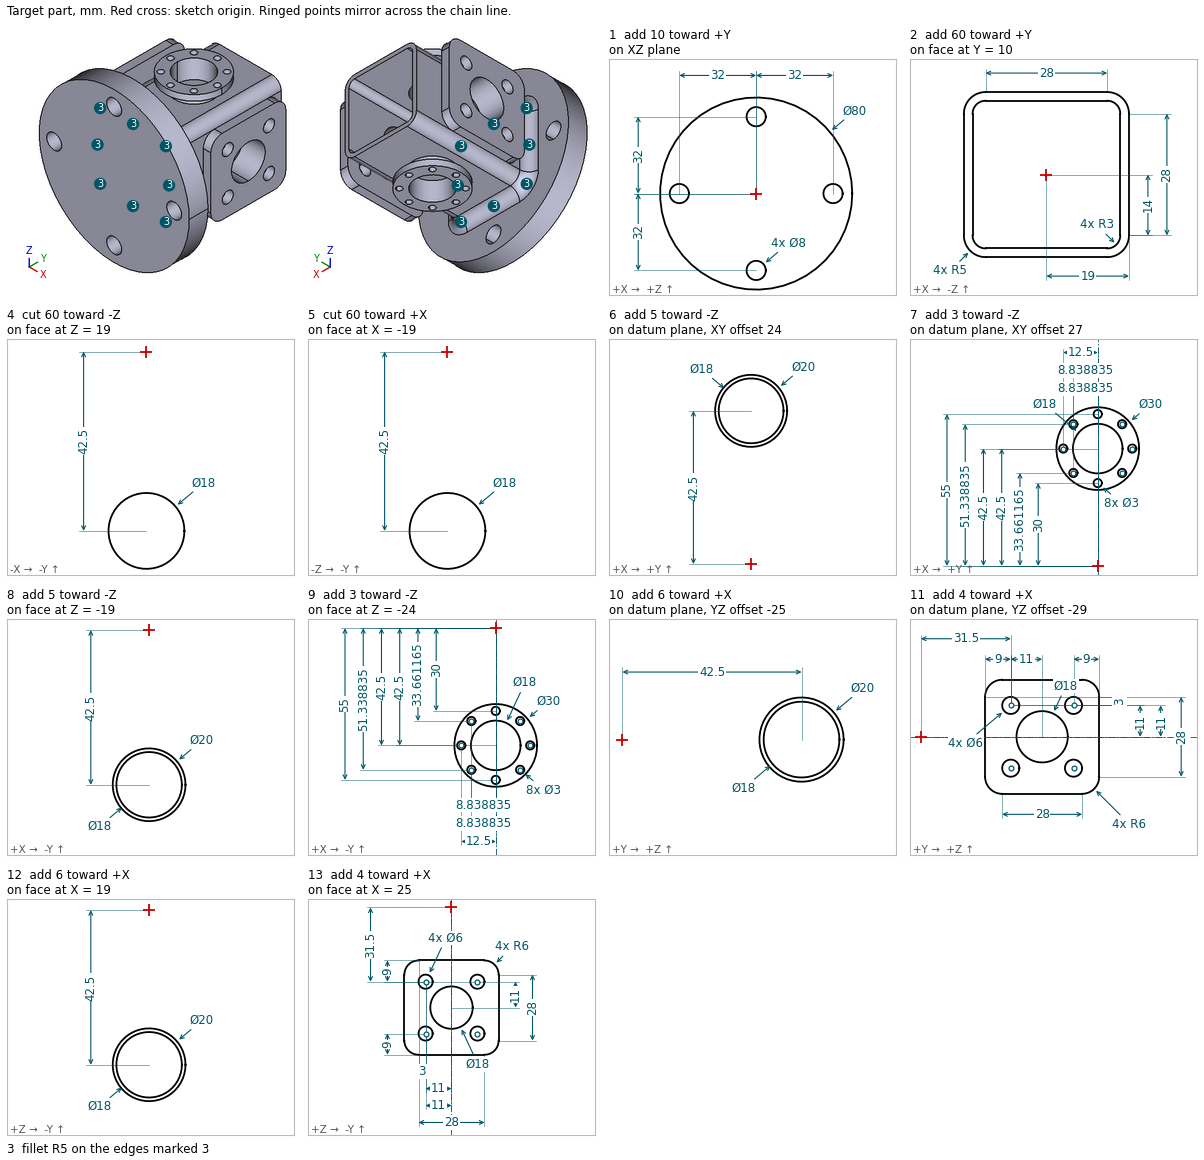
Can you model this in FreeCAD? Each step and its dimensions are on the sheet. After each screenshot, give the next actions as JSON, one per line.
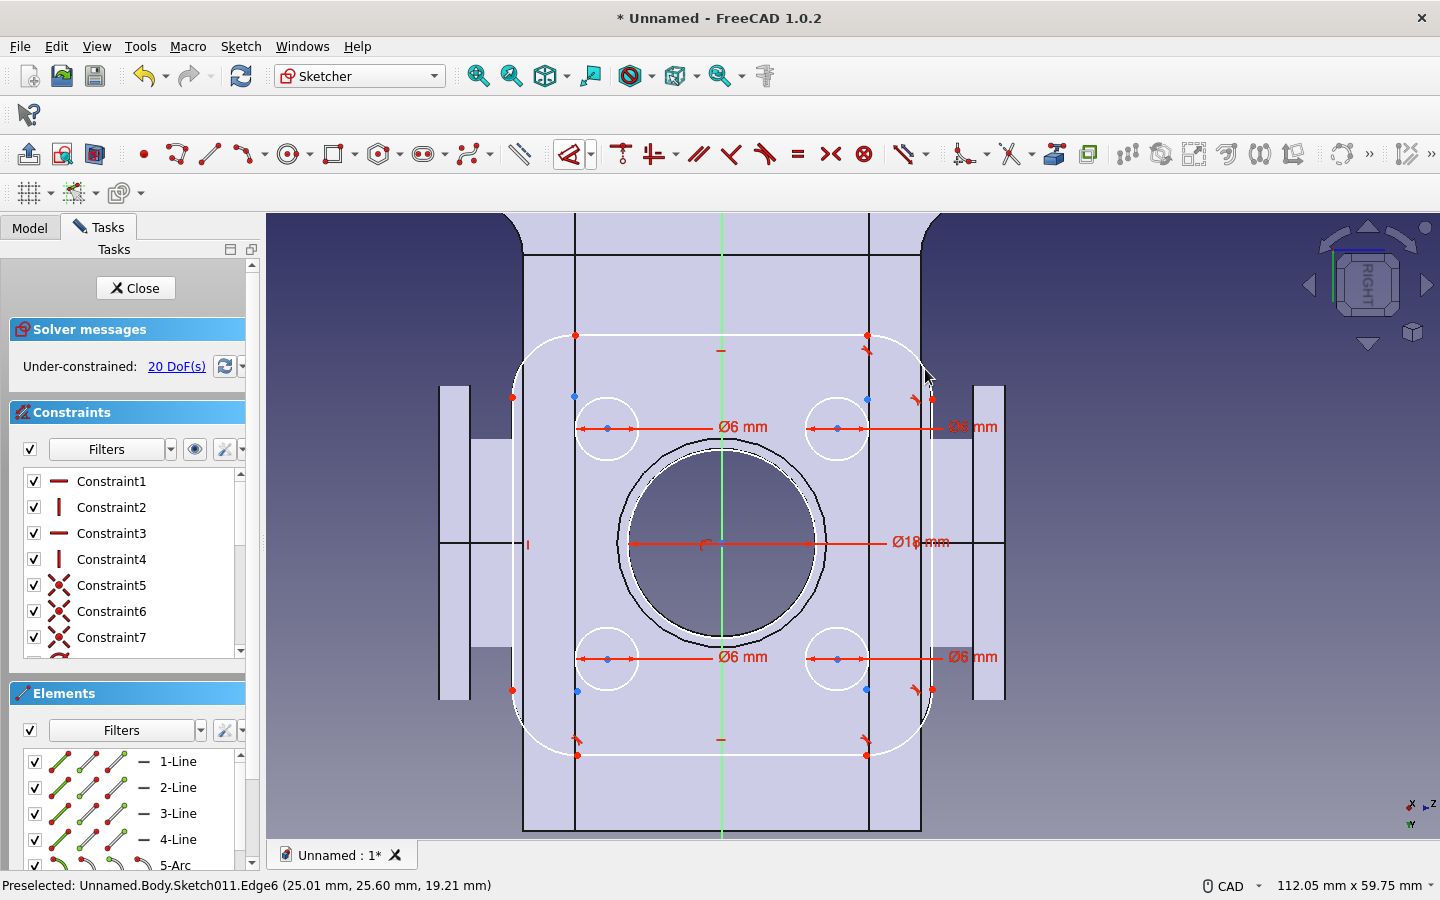
{"action": "left_click", "coordinate": [780, 335]}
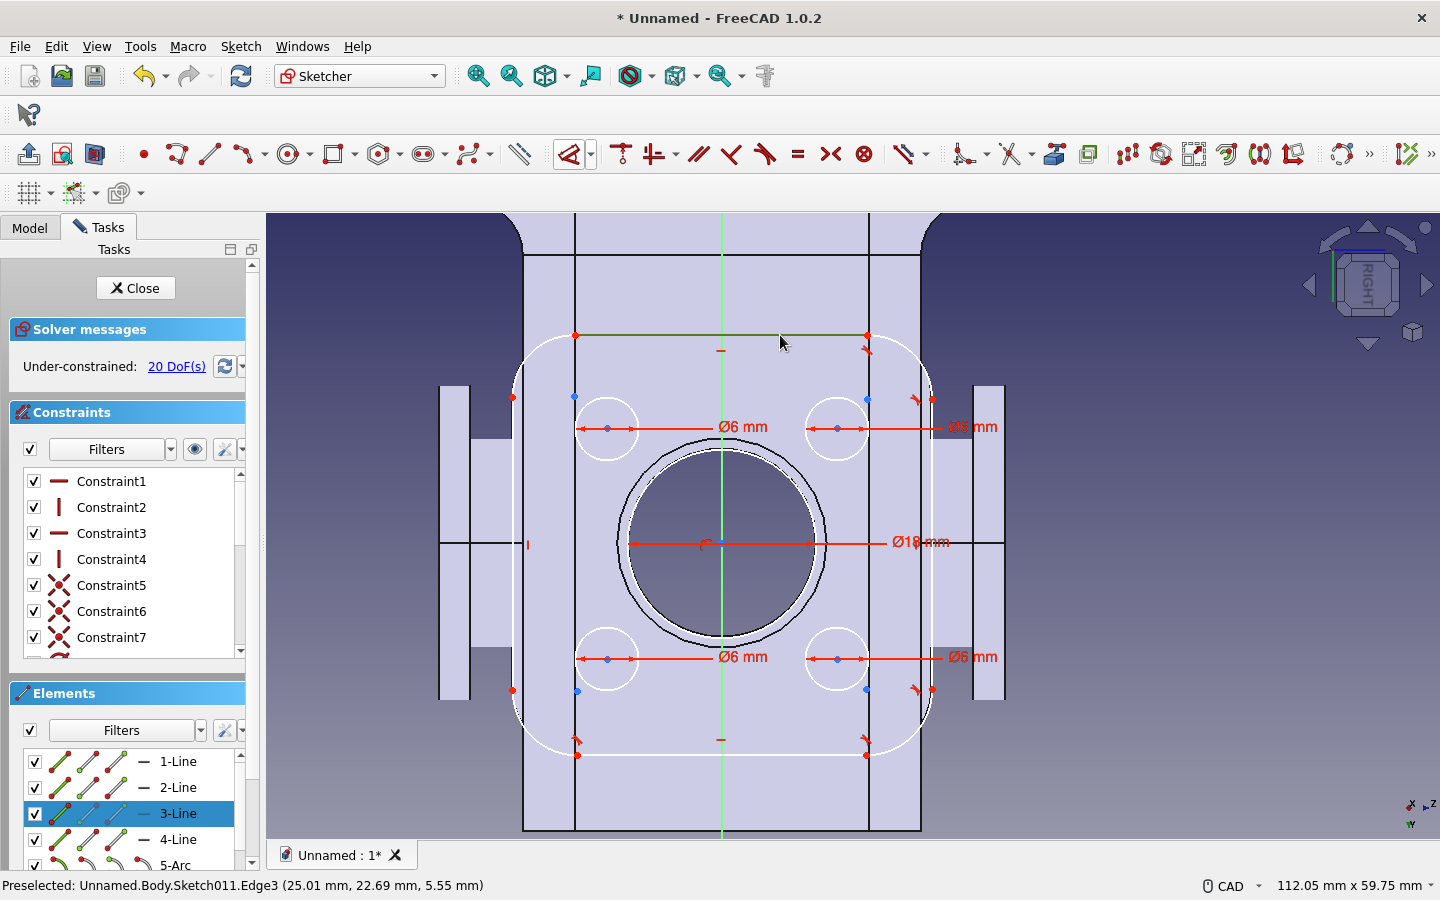
{"action": "left_click", "coordinate": [547, 342]}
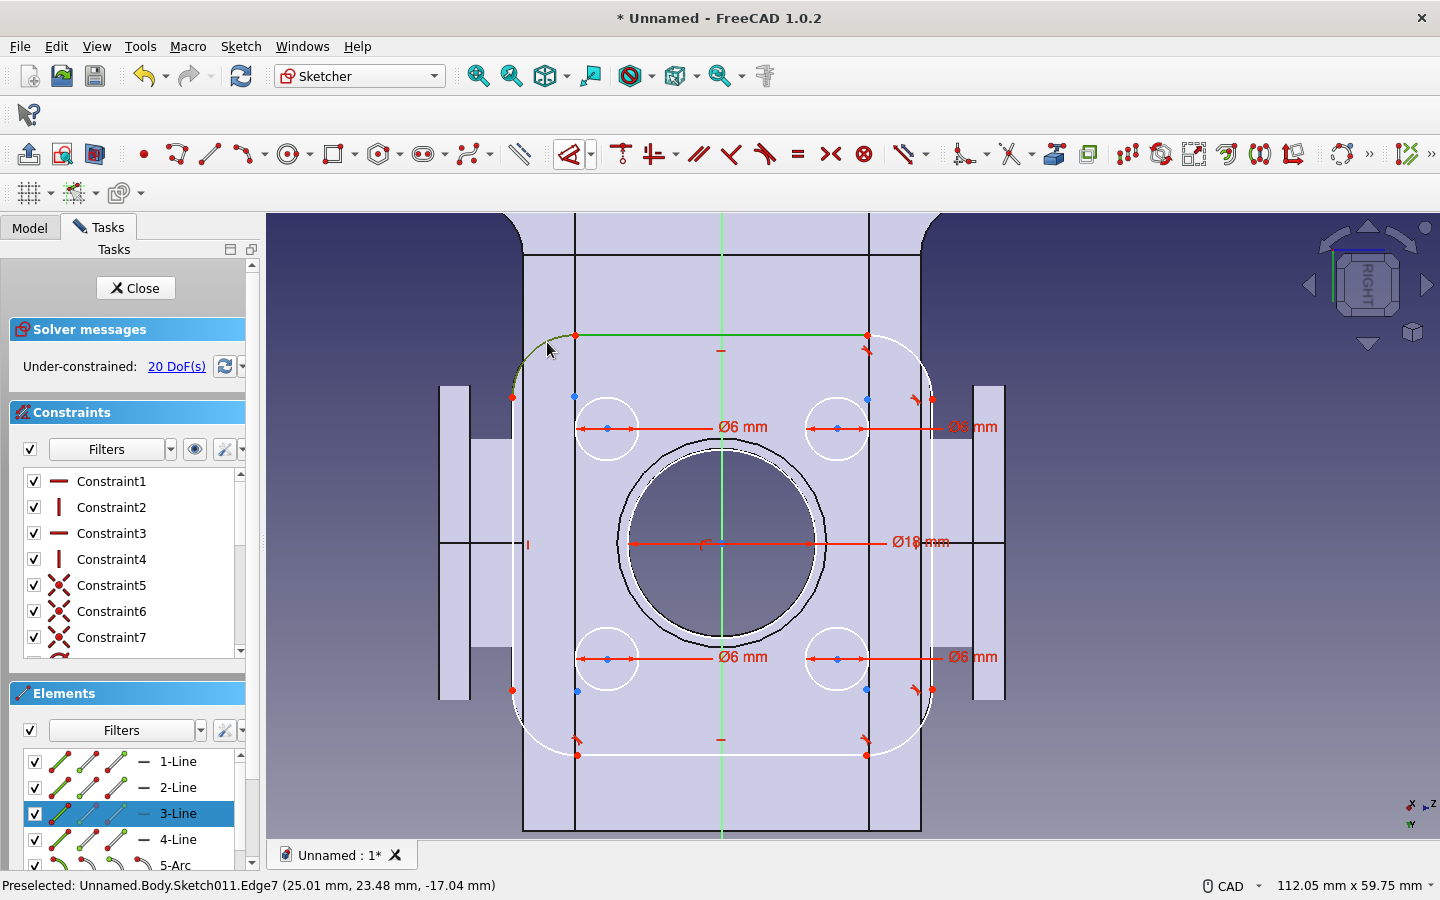
{"action": "key", "text": "t"}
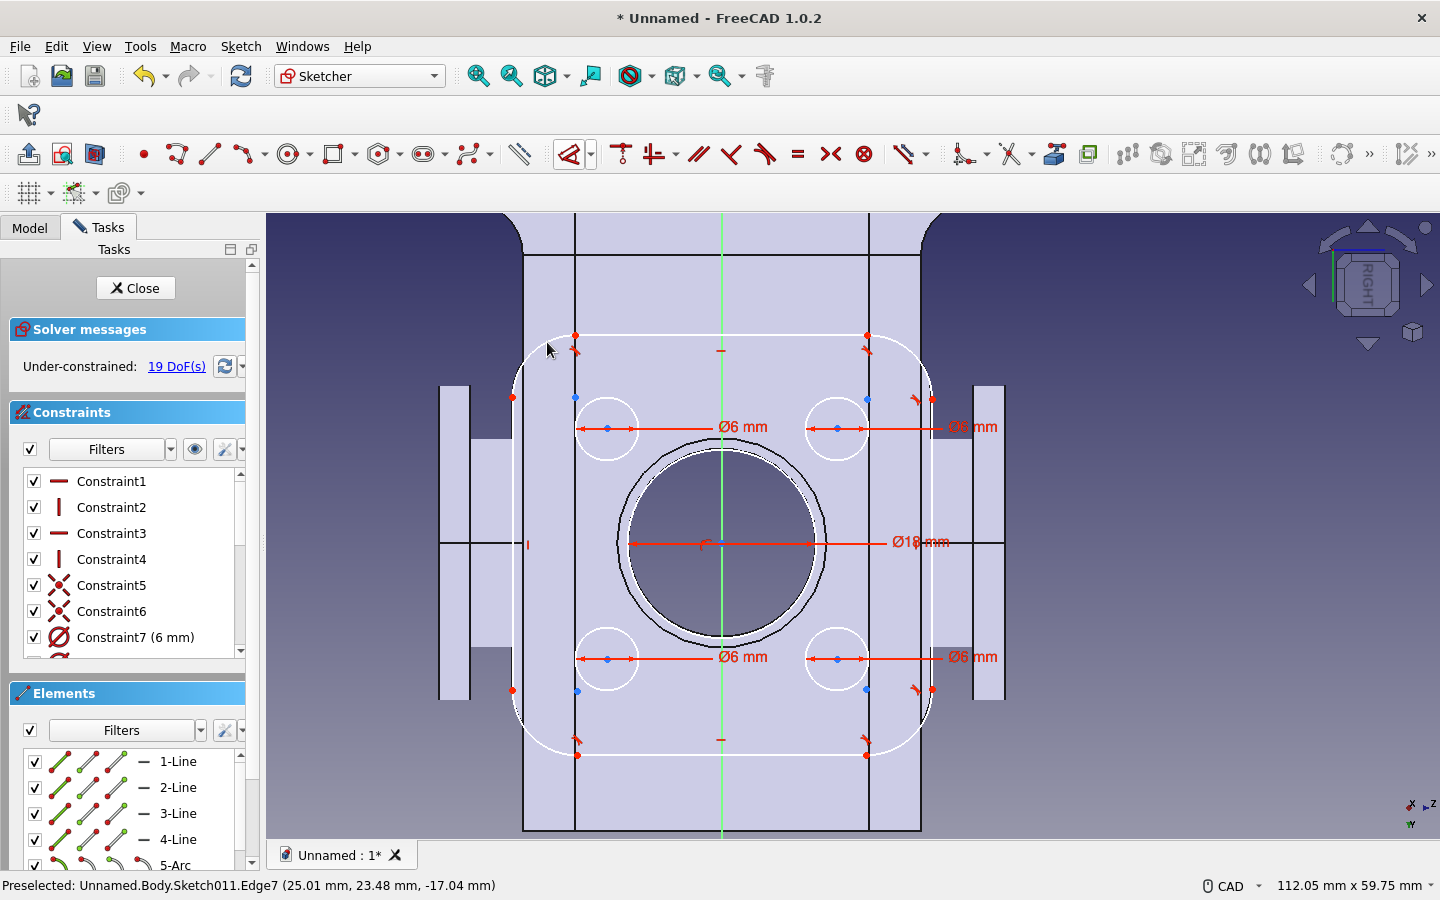
{"action": "left_click", "coordinate": [513, 486]}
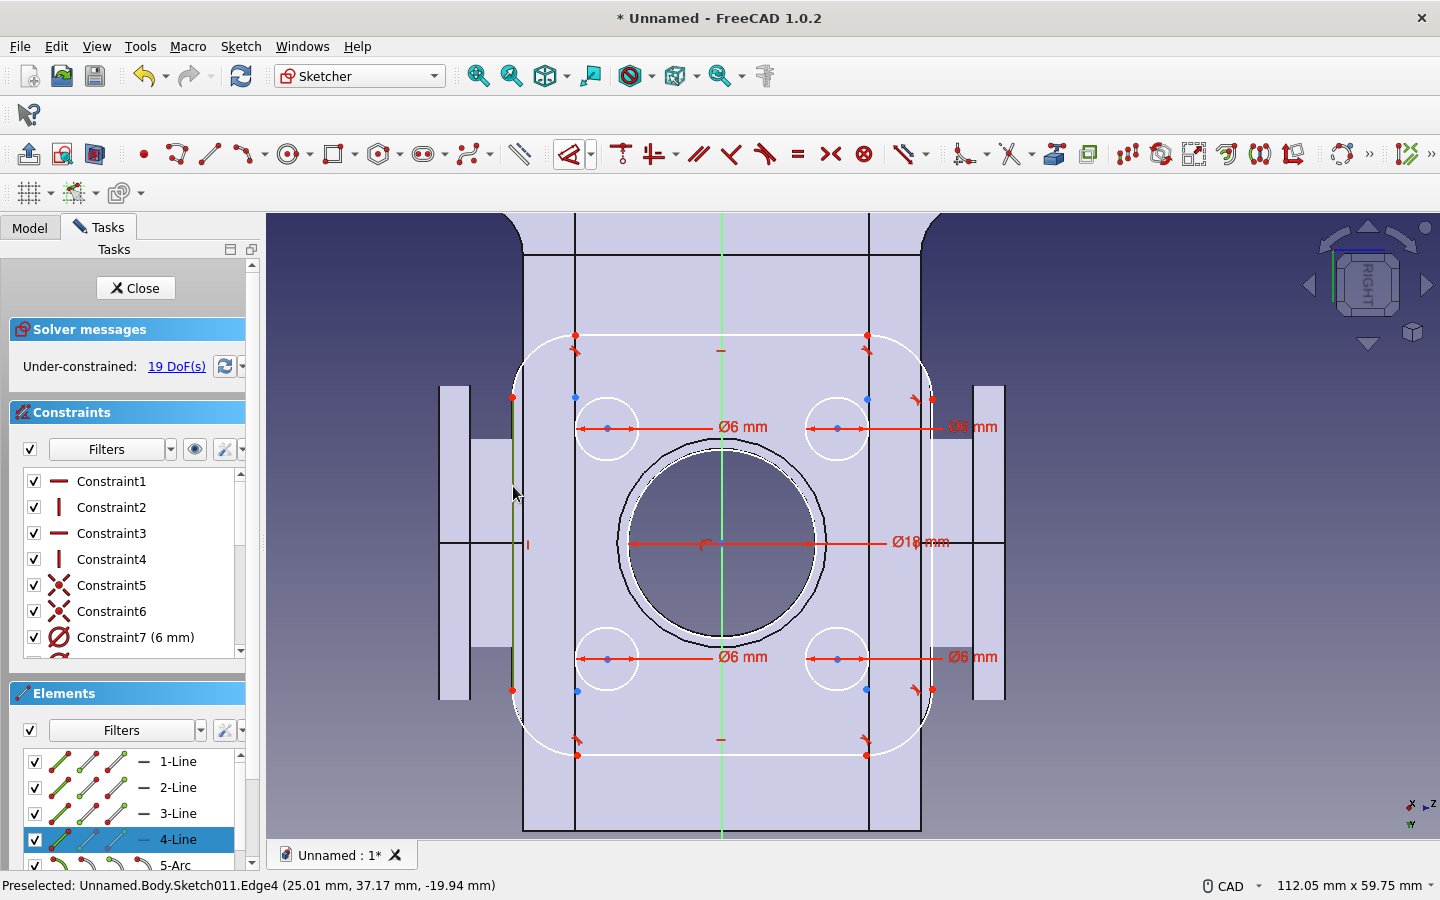
{"action": "left_click", "coordinate": [547, 342]}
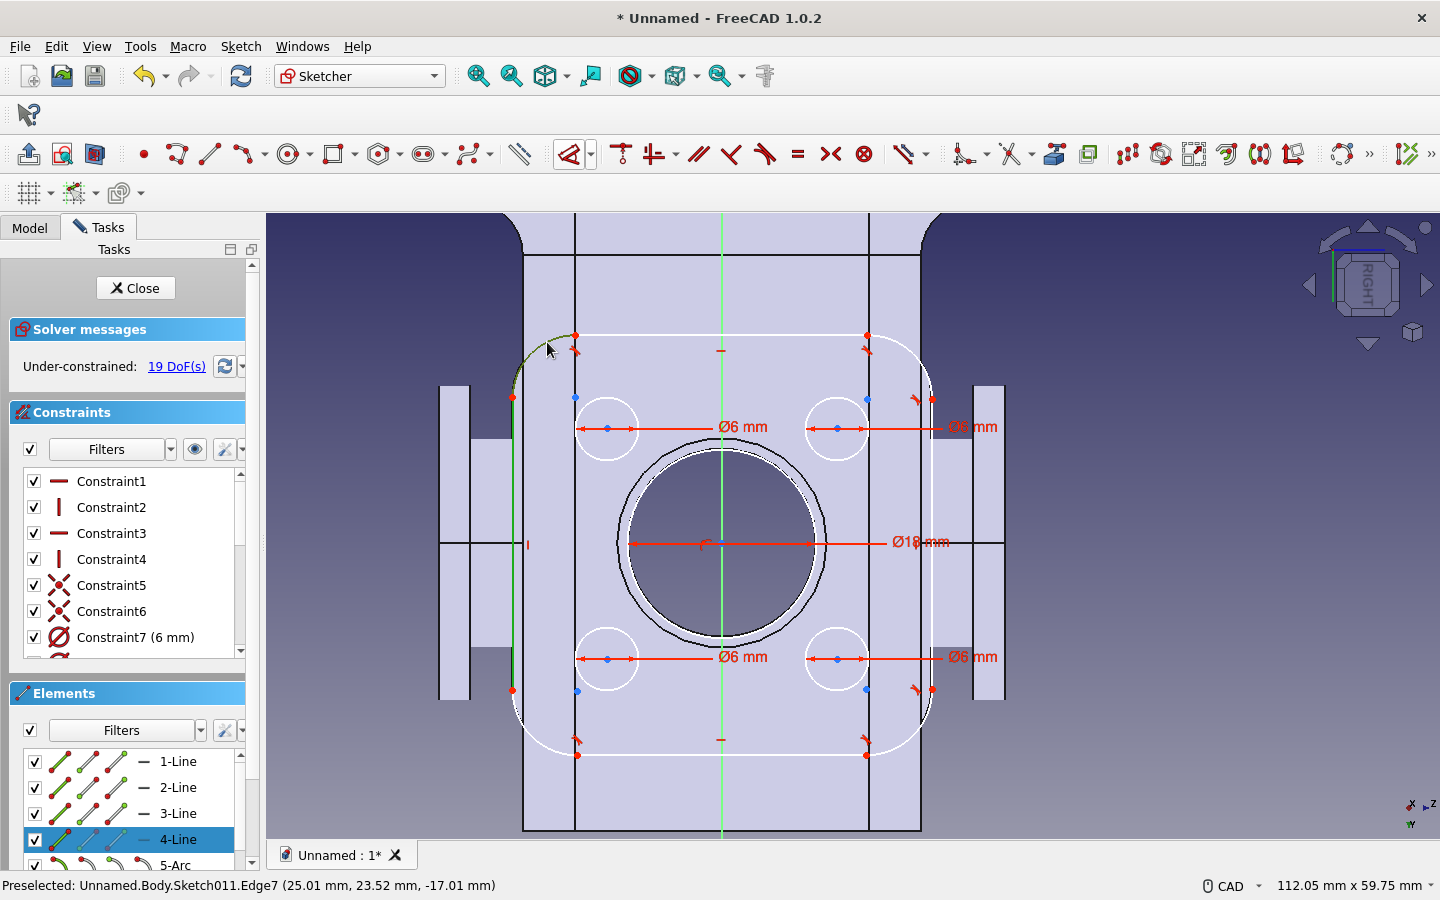
{"action": "key", "text": "t"}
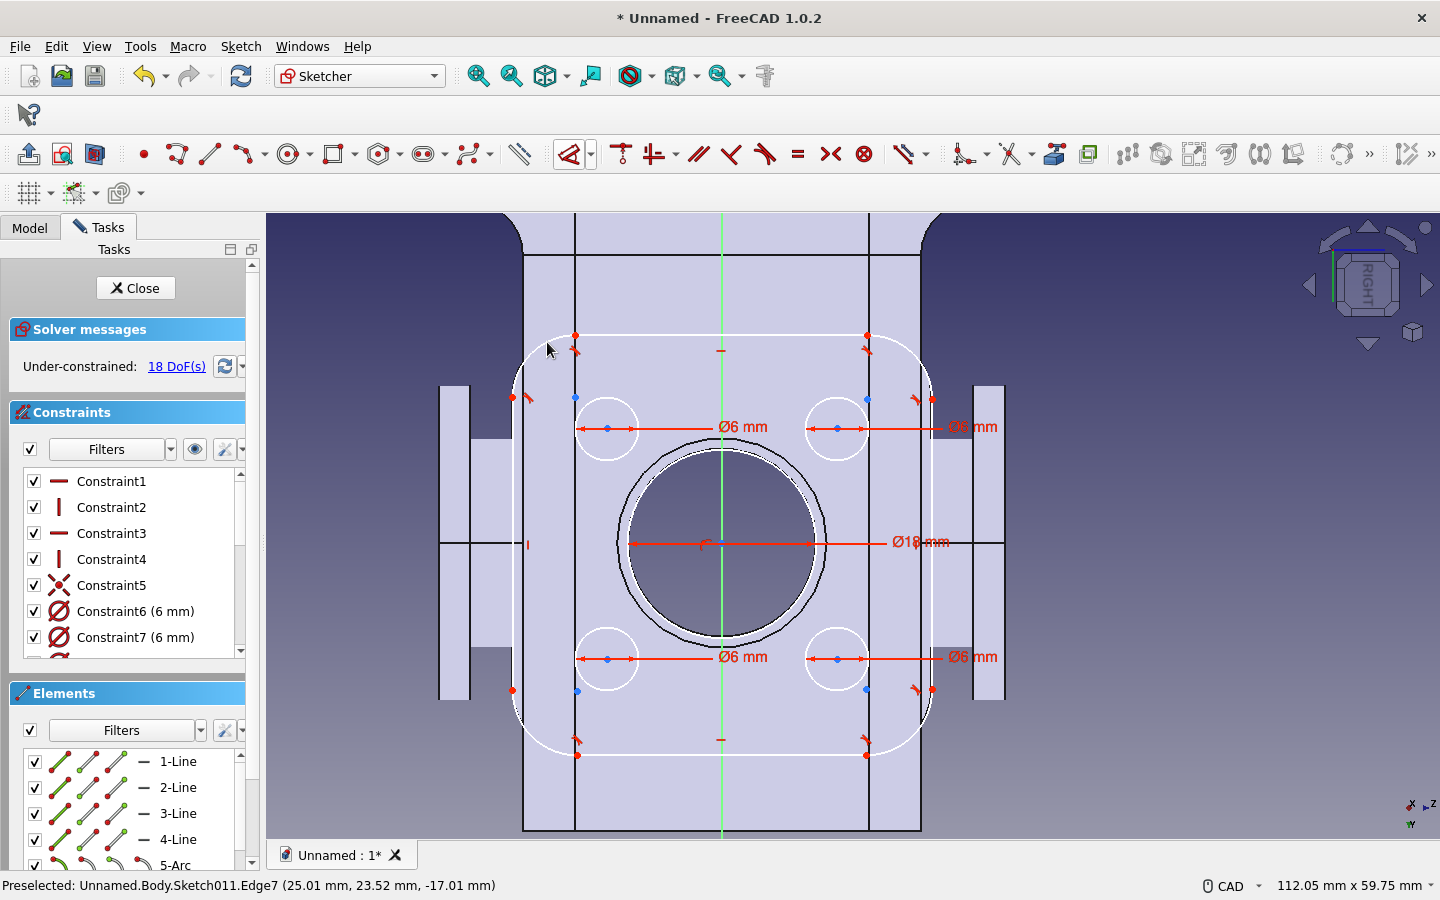
{"action": "left_click", "coordinate": [513, 486]}